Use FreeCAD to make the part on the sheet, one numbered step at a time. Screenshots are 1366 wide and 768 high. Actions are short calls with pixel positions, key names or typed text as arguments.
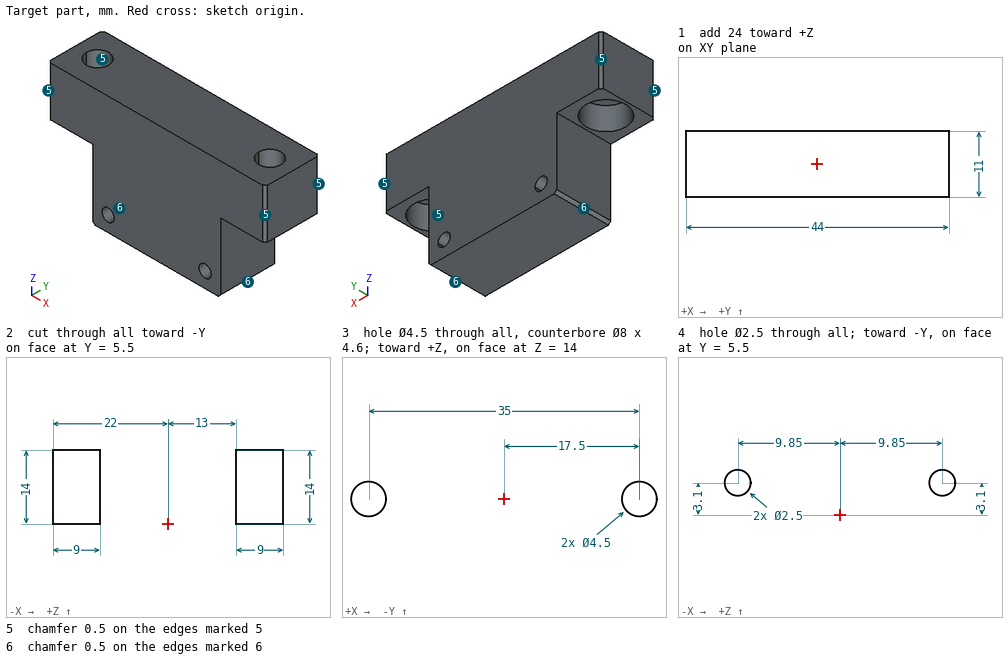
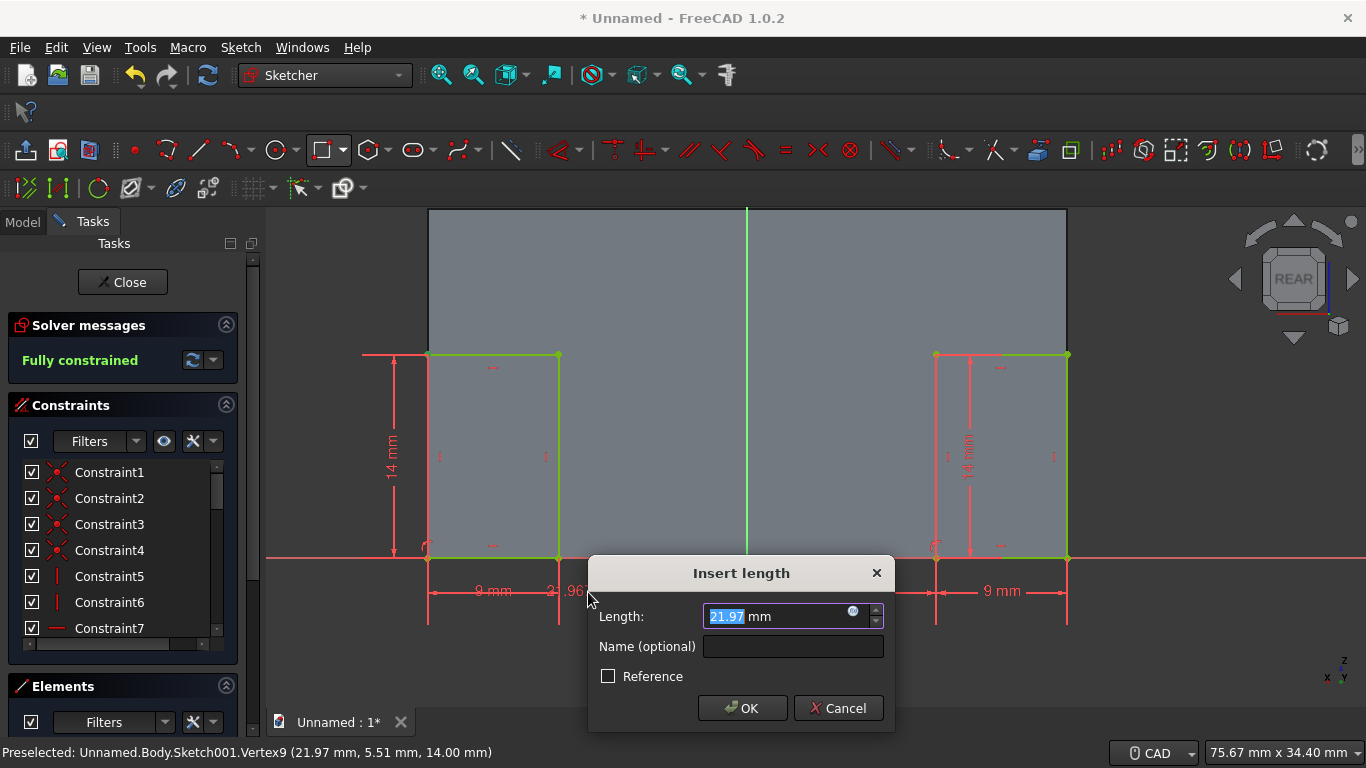
text(22)
key(Return)
key(Escape)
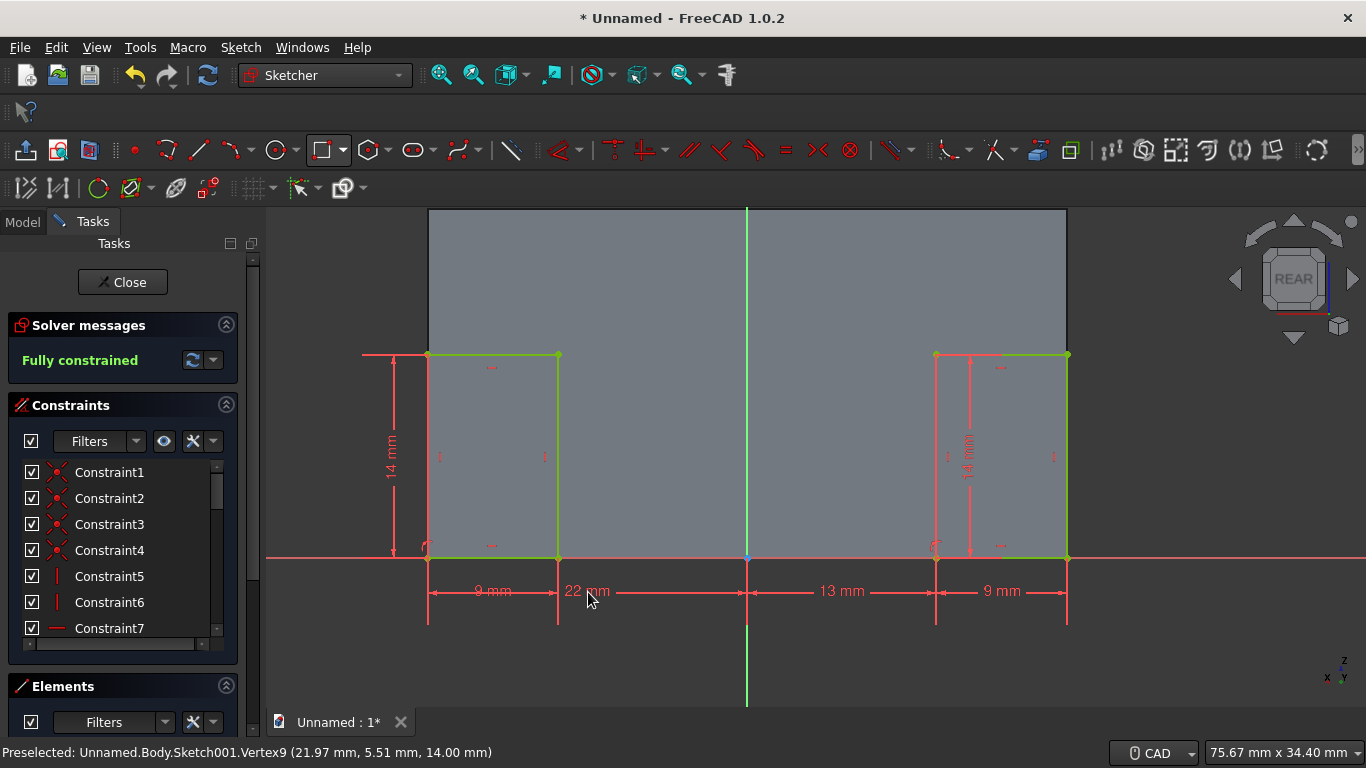
click(123, 282)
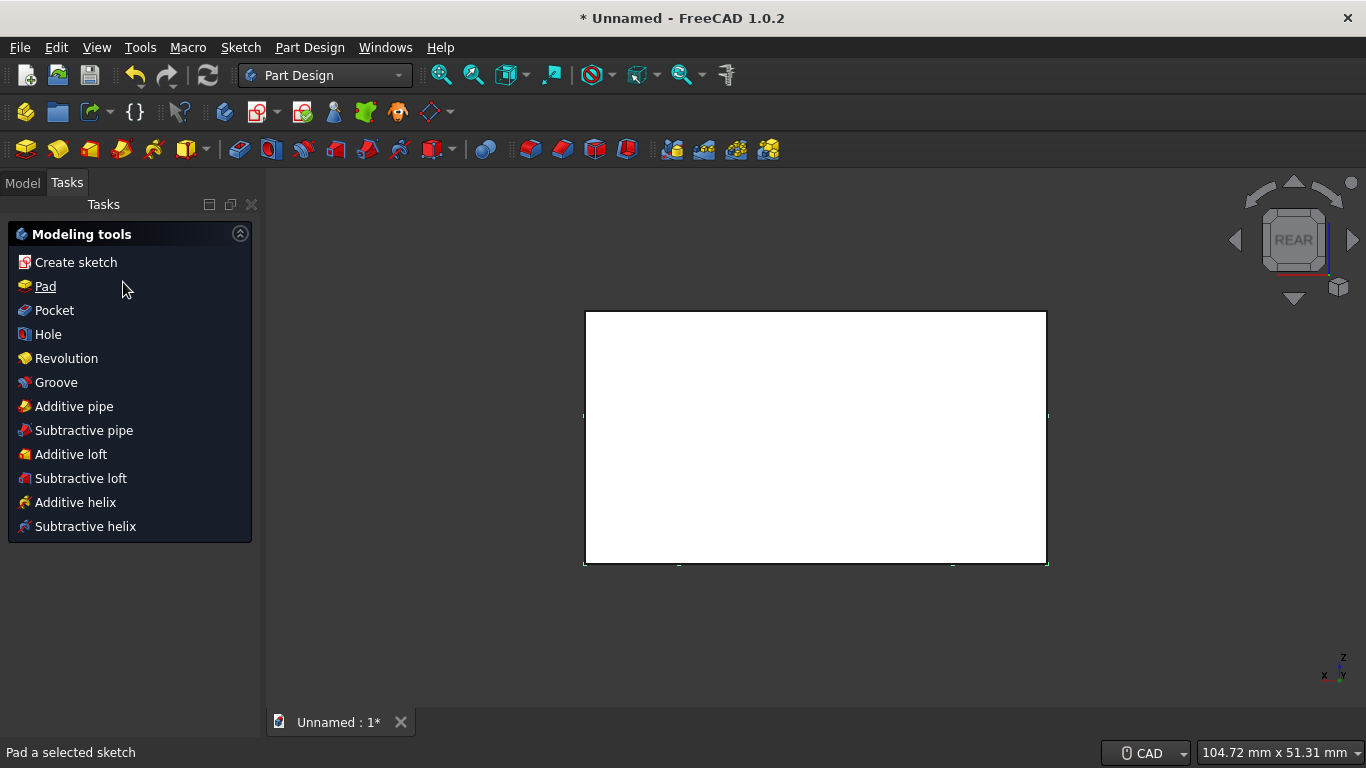
click(240, 150)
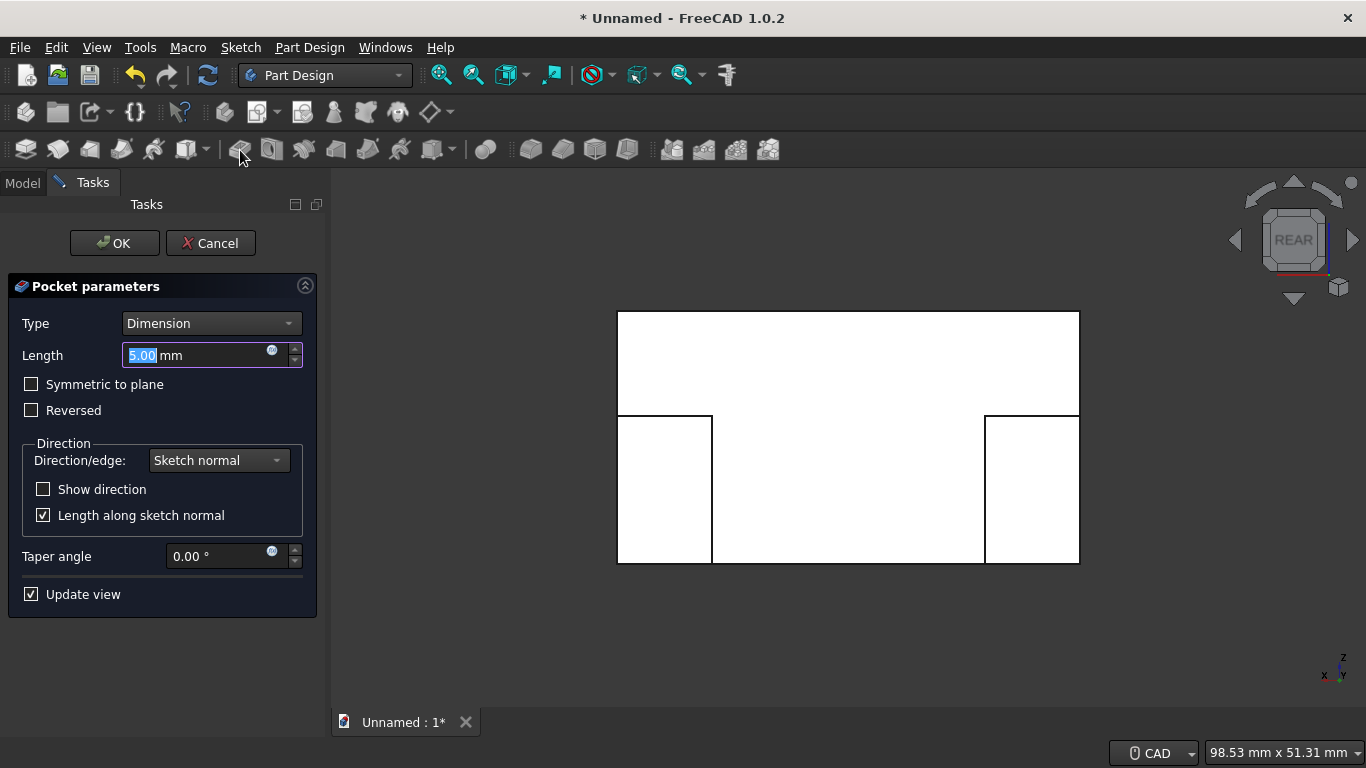
click(212, 324)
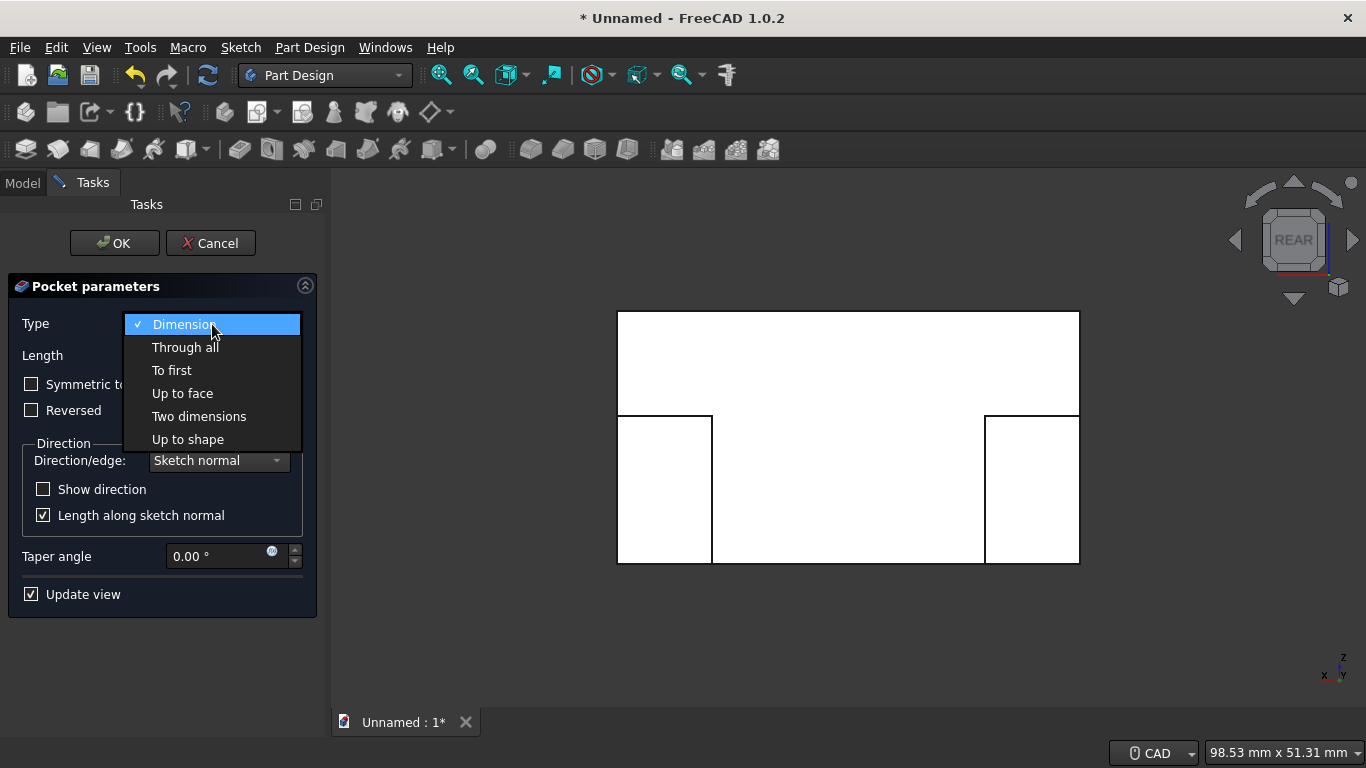
click(212, 348)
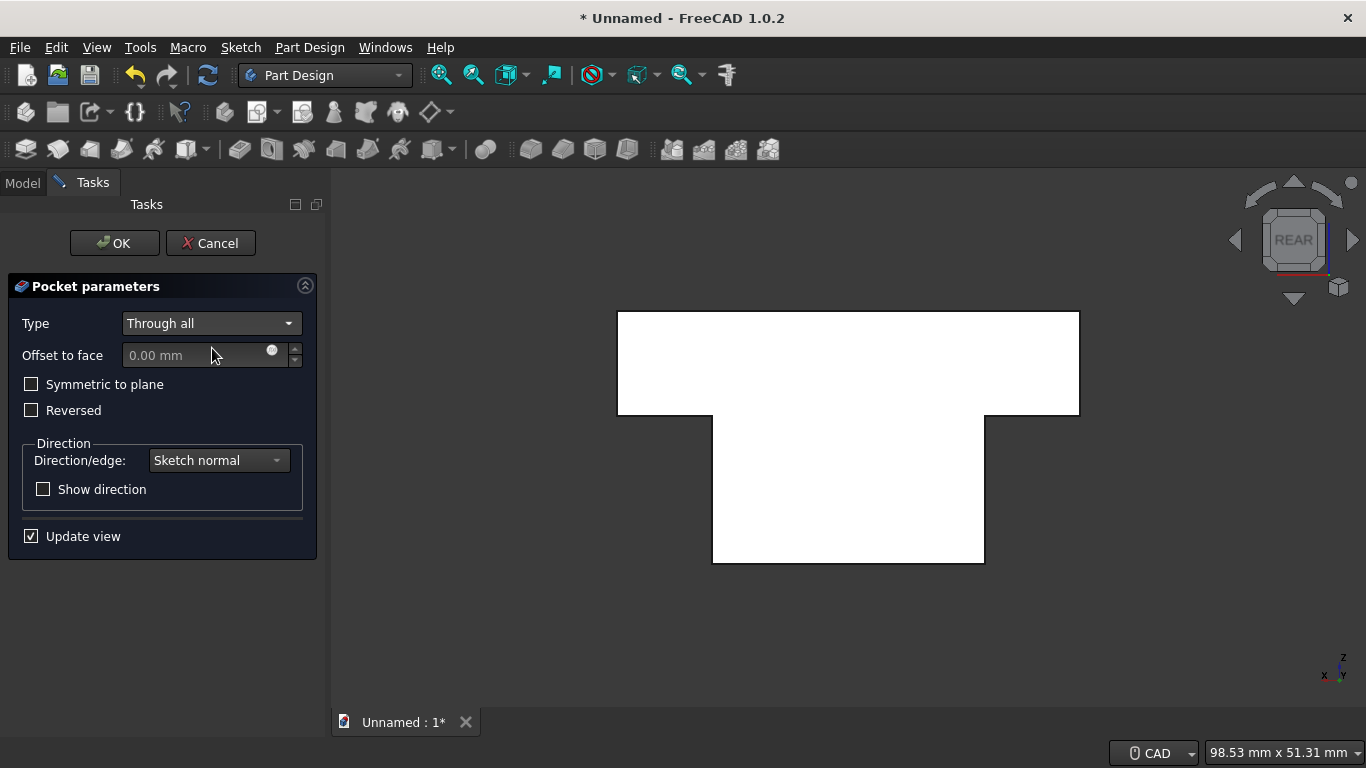
click(115, 243)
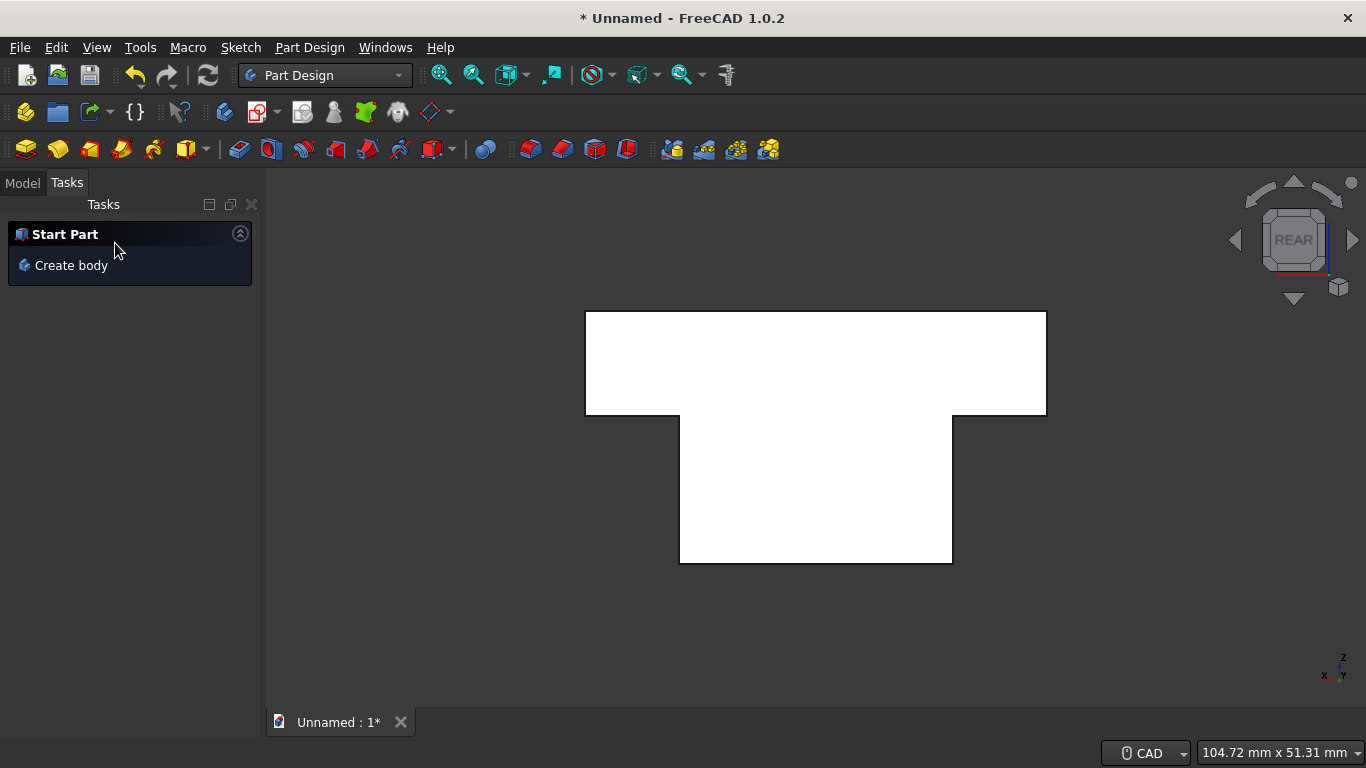
key(5)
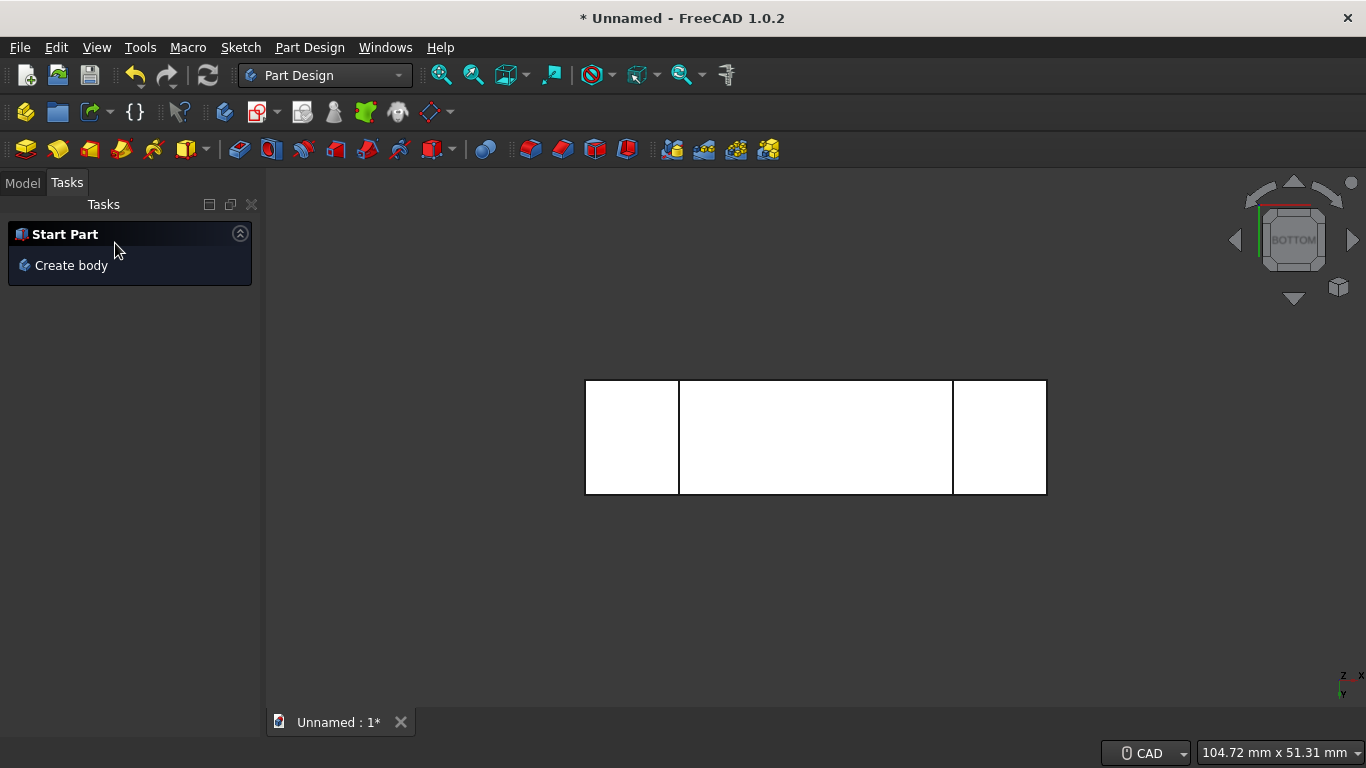
click(442, 76)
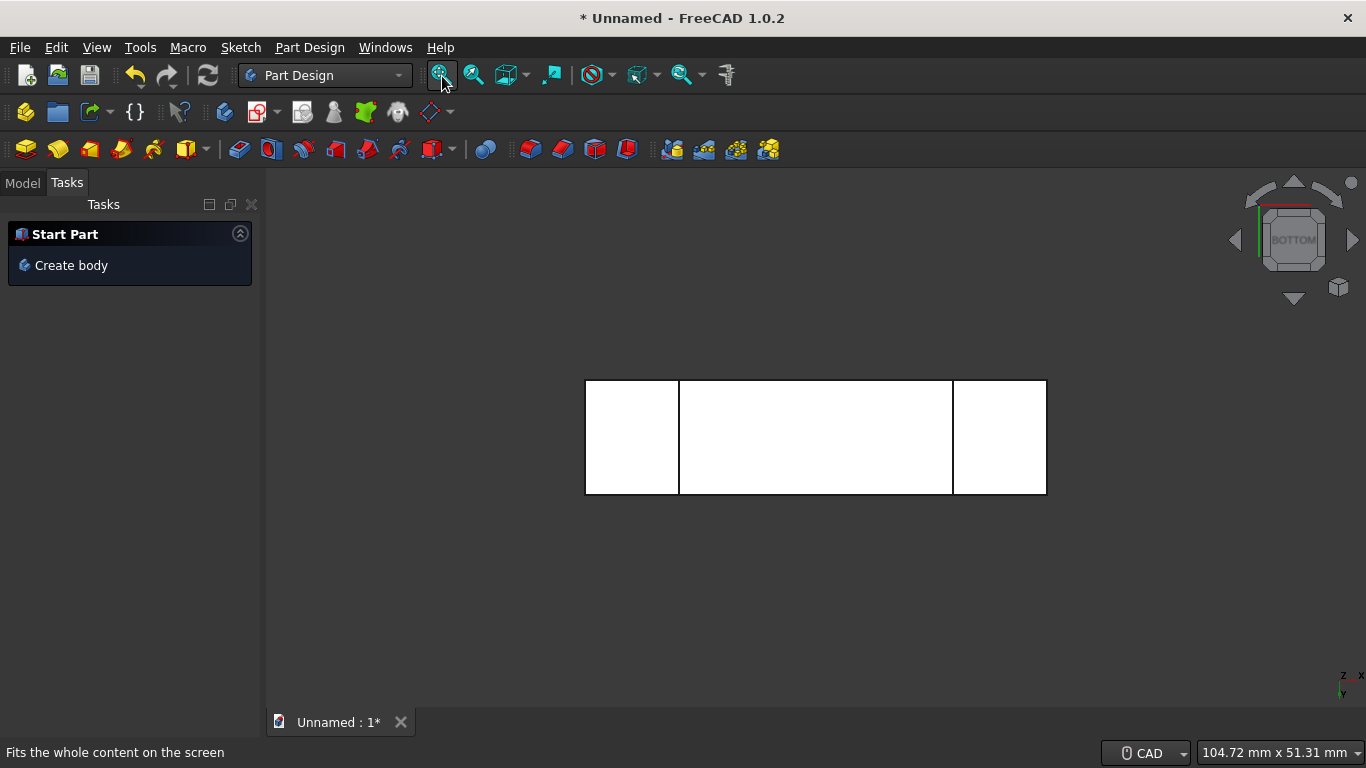
click(1000, 436)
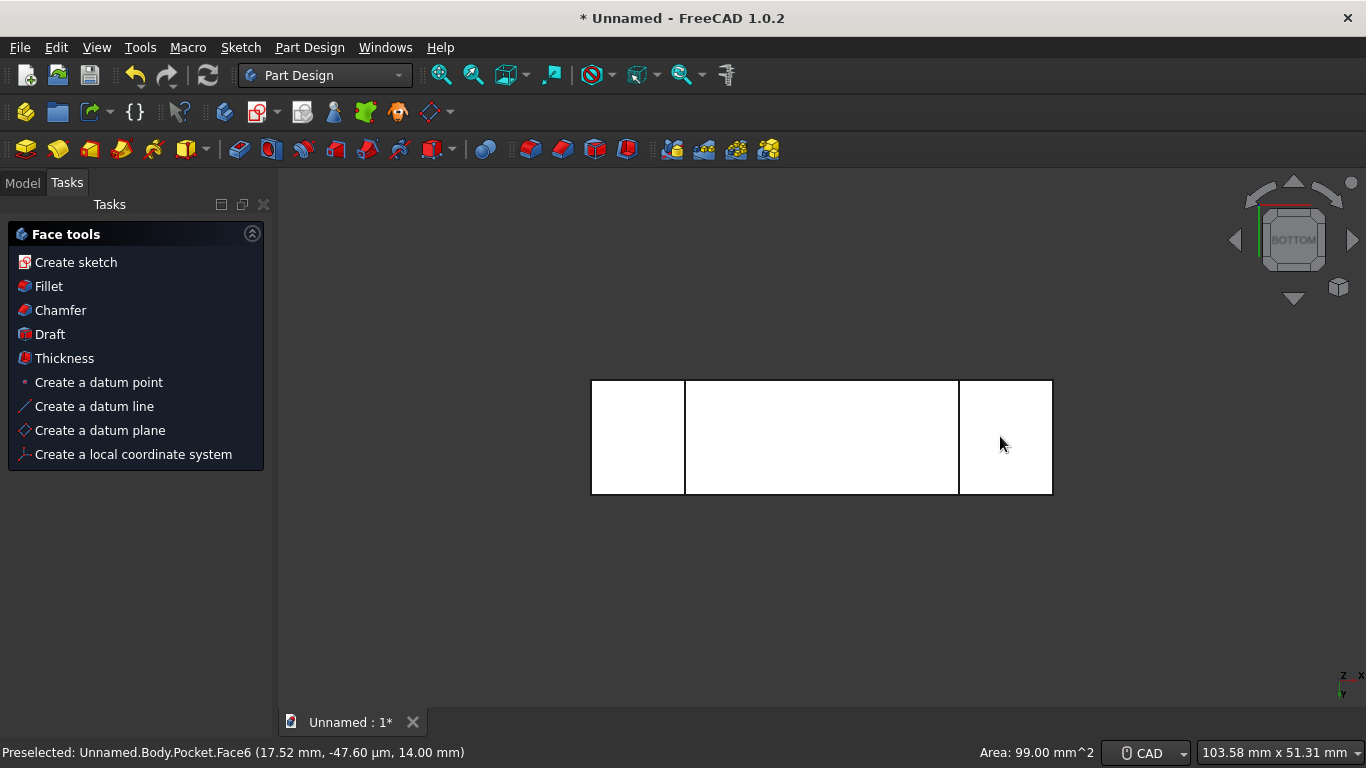
click(258, 112)